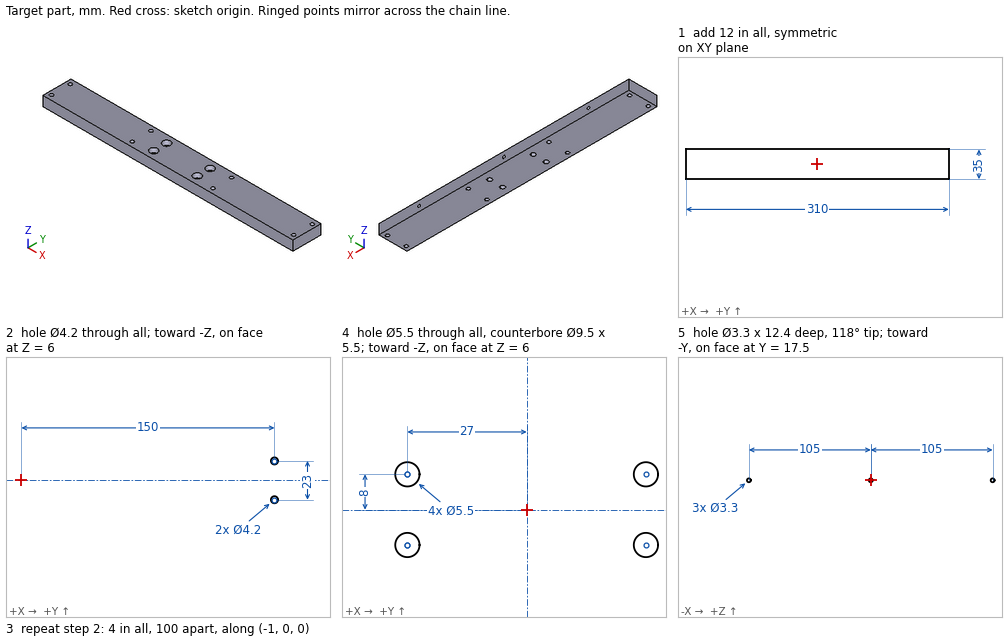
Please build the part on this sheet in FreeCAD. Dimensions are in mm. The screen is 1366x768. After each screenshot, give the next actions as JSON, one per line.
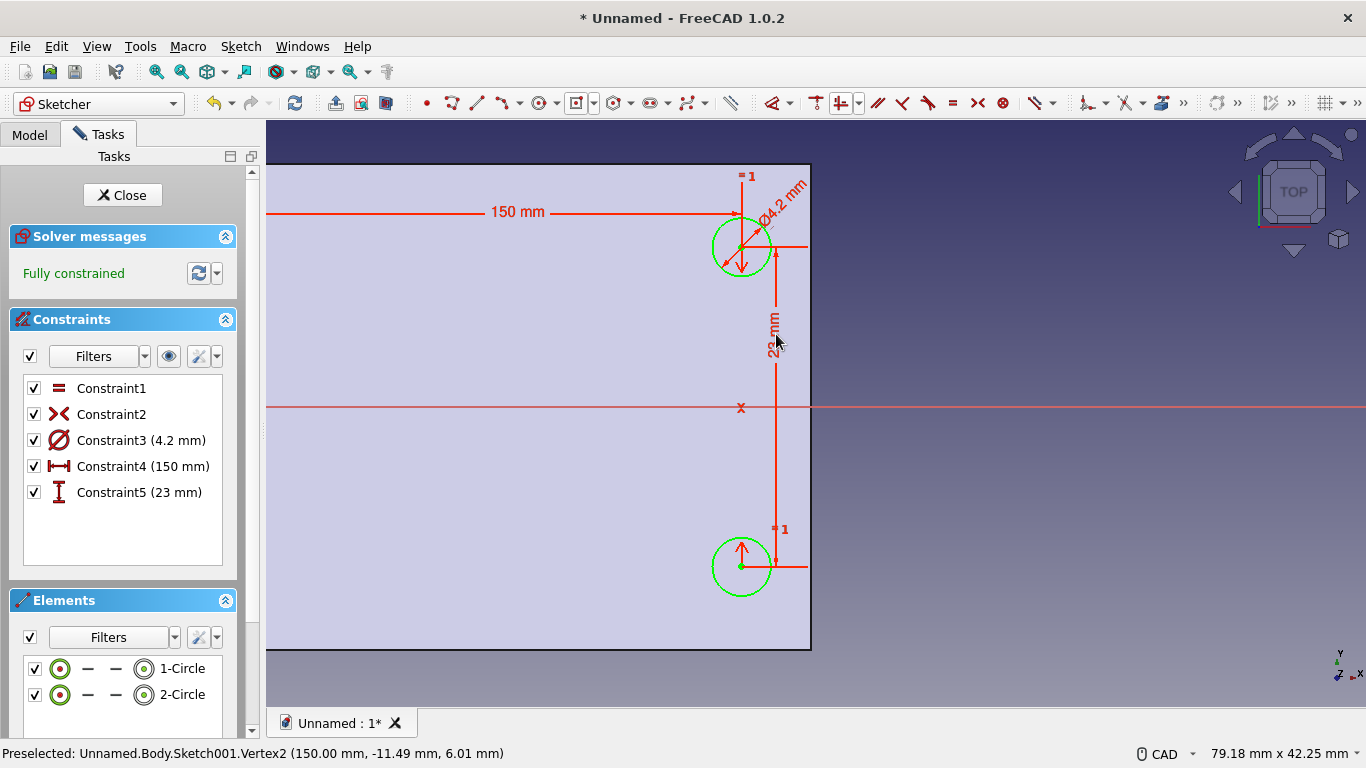
{"action": "left_click", "coordinate": [123, 195]}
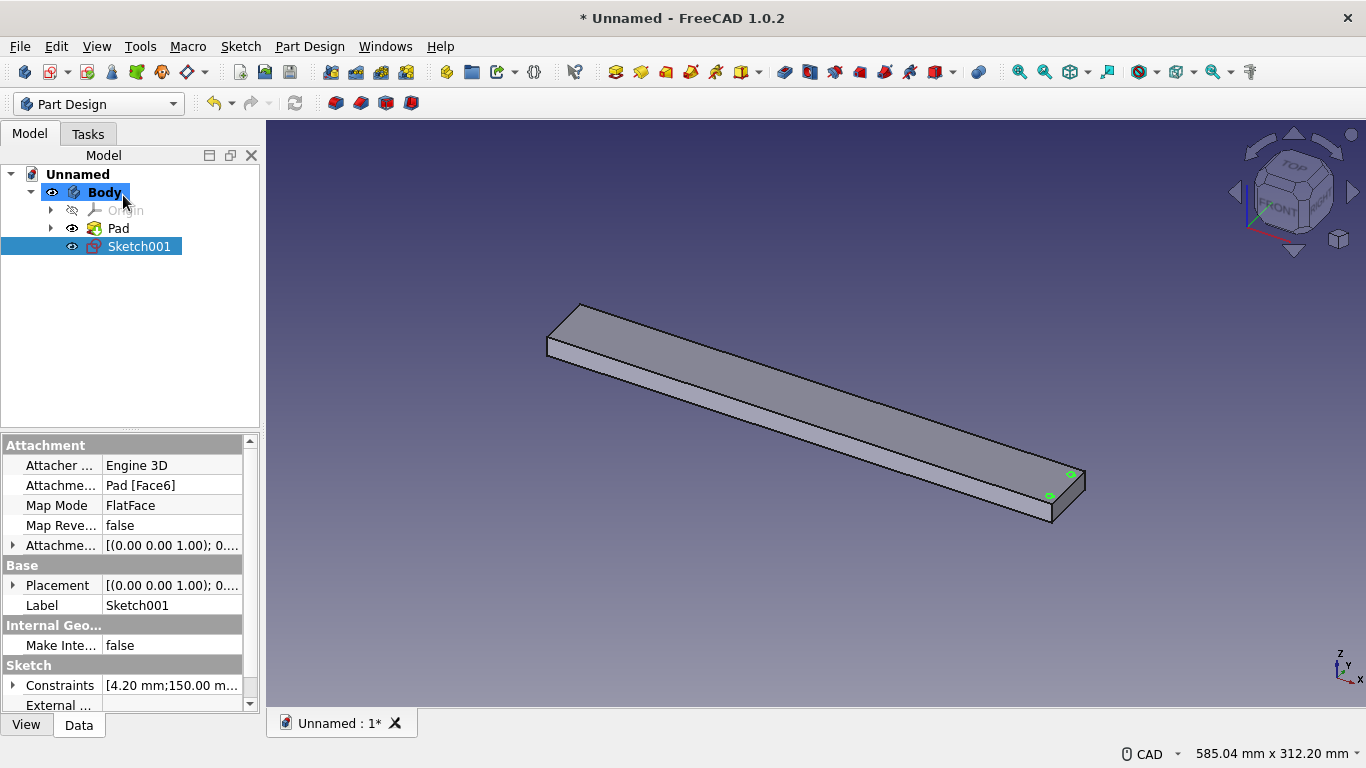
{"action": "left_click", "coordinate": [810, 72]}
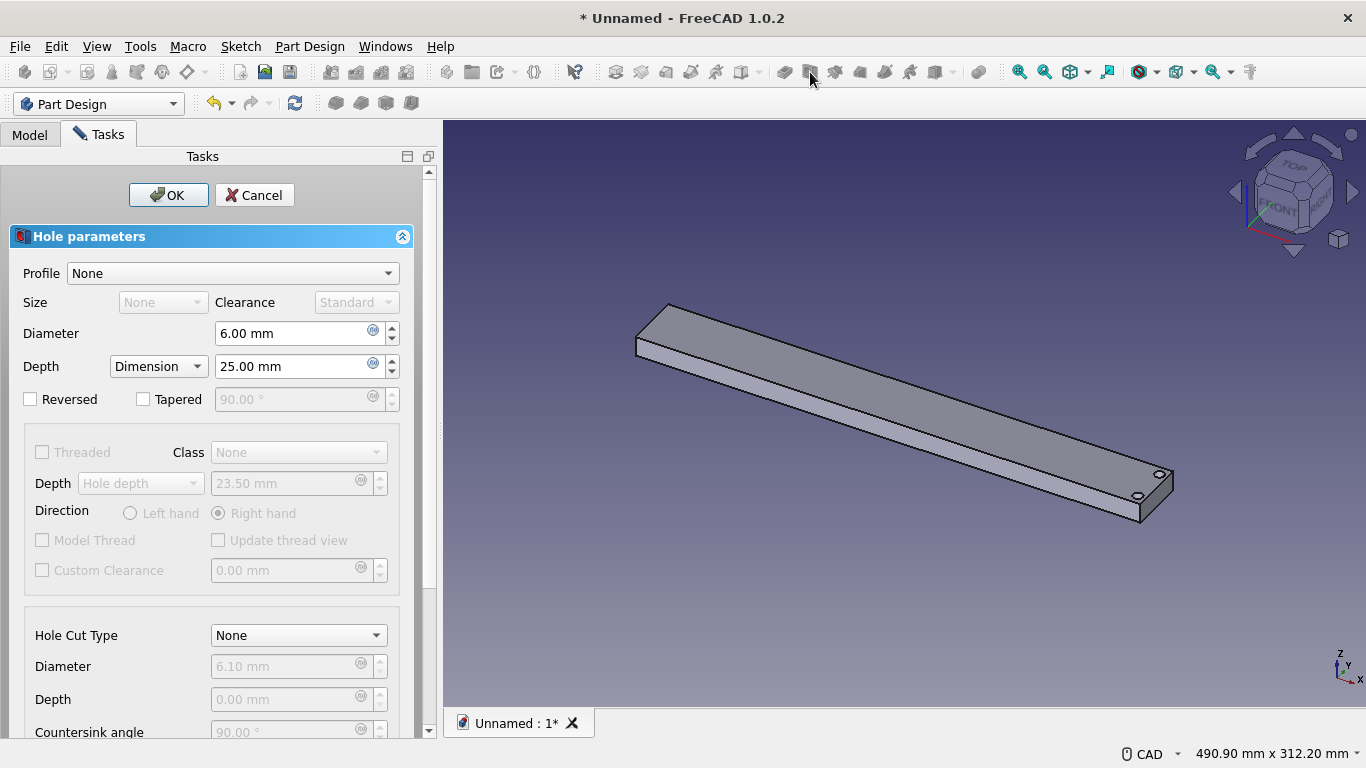
{"action": "triple_click", "coordinate": [300, 334]}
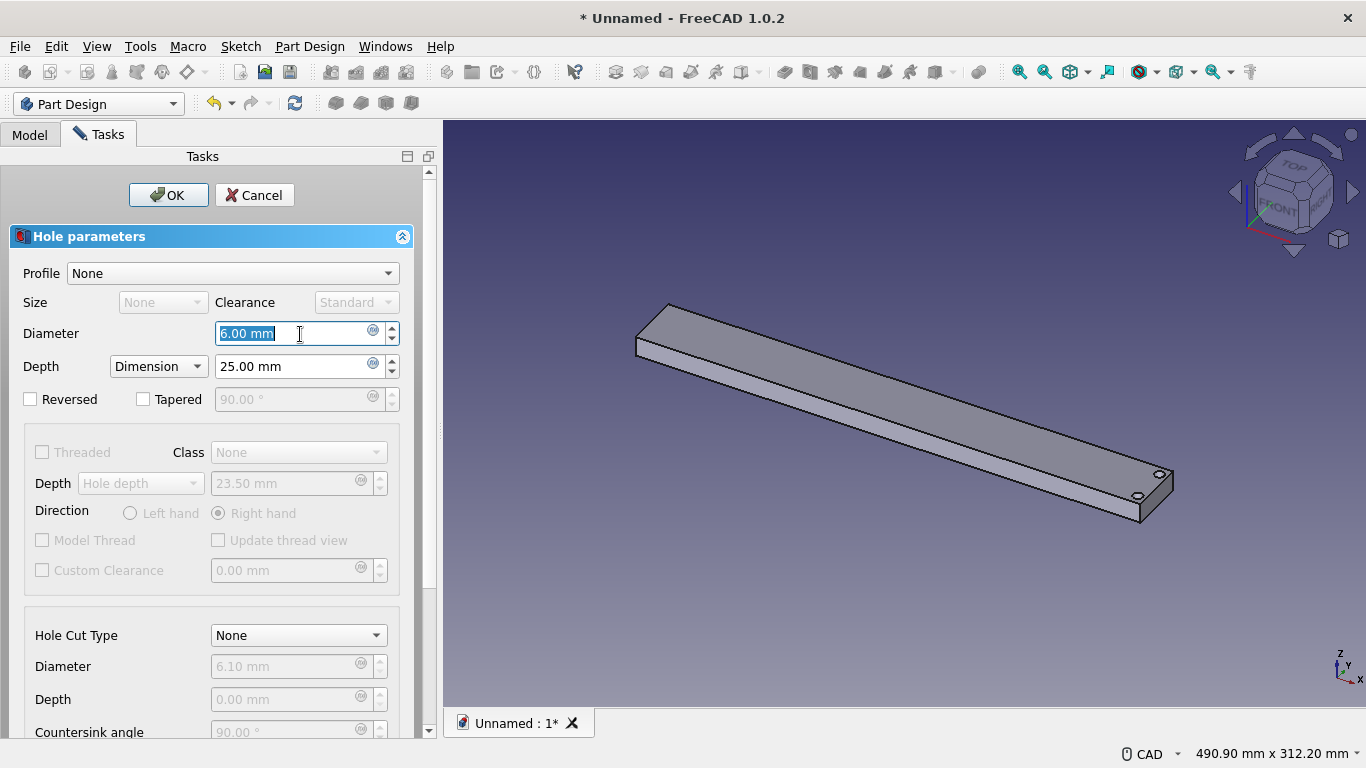
{"action": "type", "text": "4.2"}
{"action": "key", "text": "Tab"}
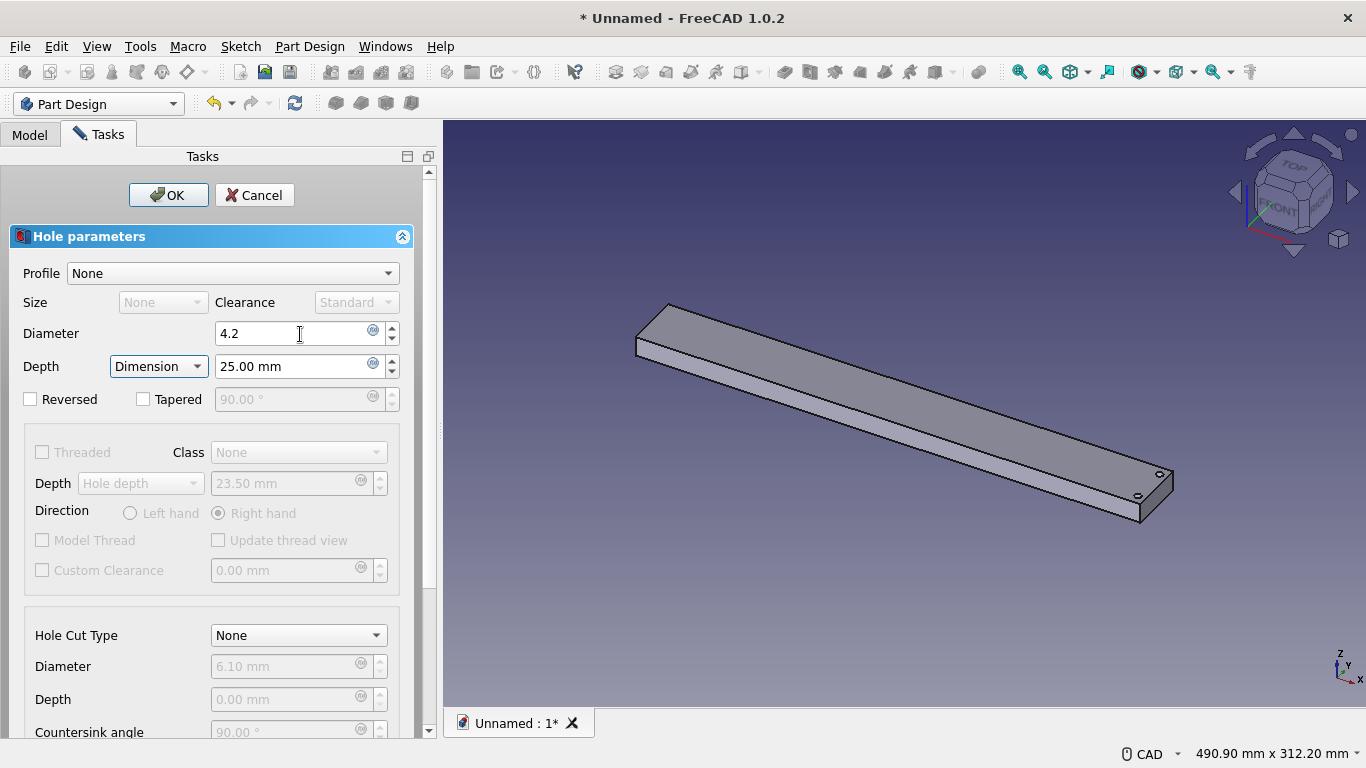
{"action": "left_click", "coordinate": [160, 366]}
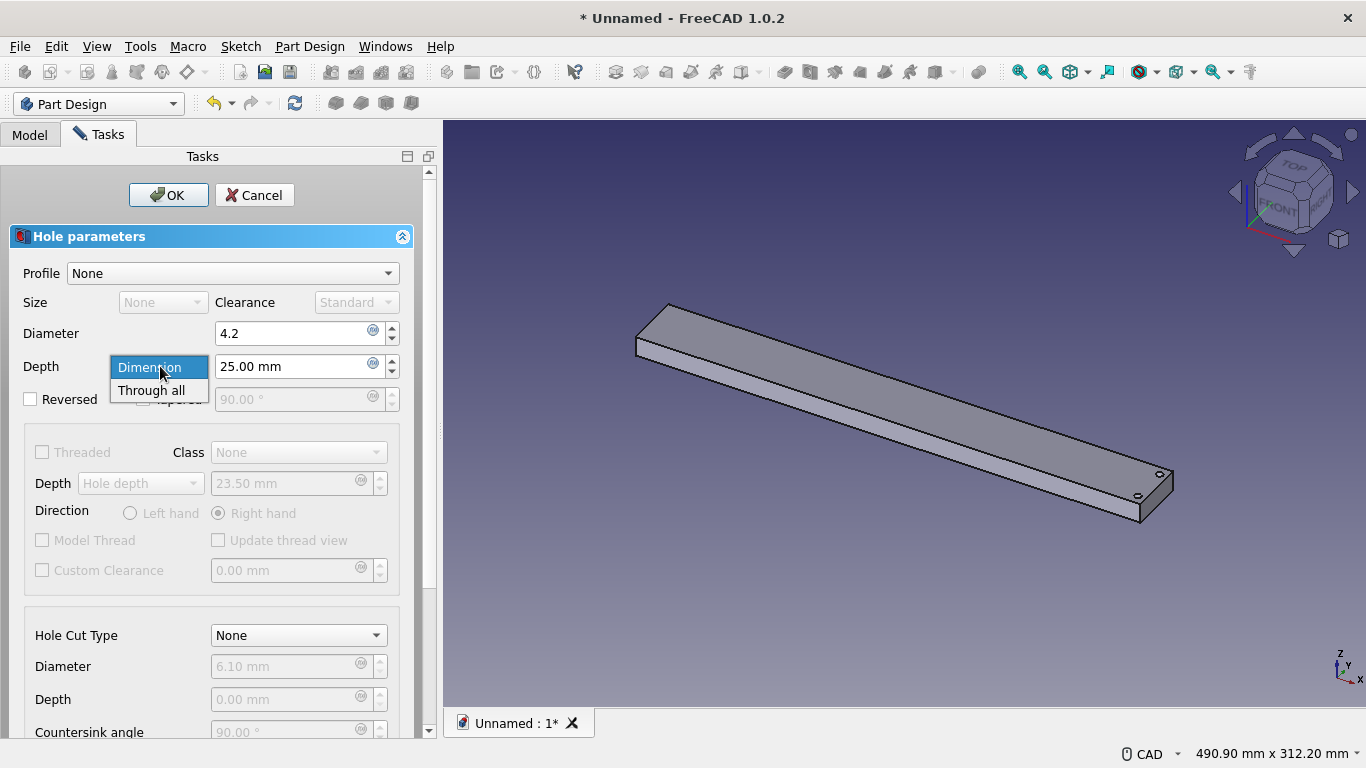
{"action": "left_click", "coordinate": [158, 390]}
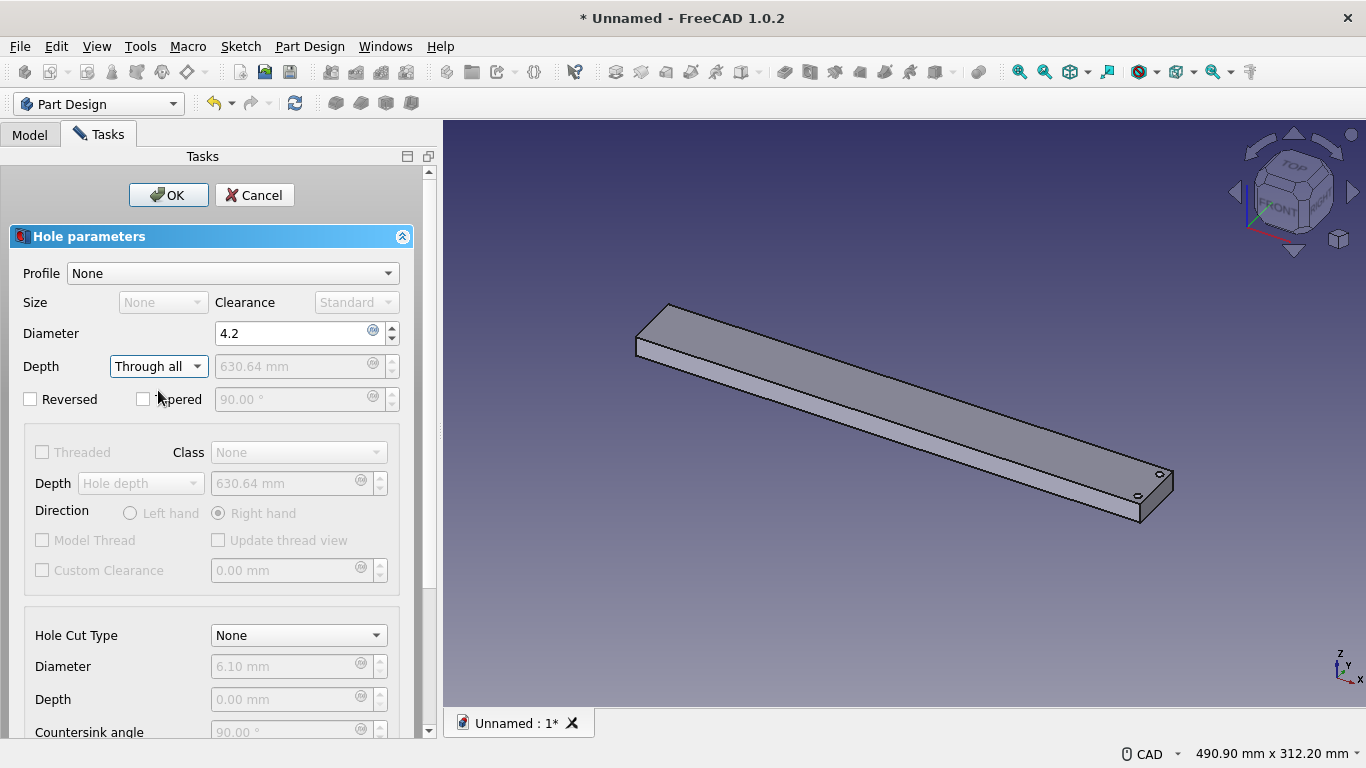
{"action": "left_click", "coordinate": [169, 195]}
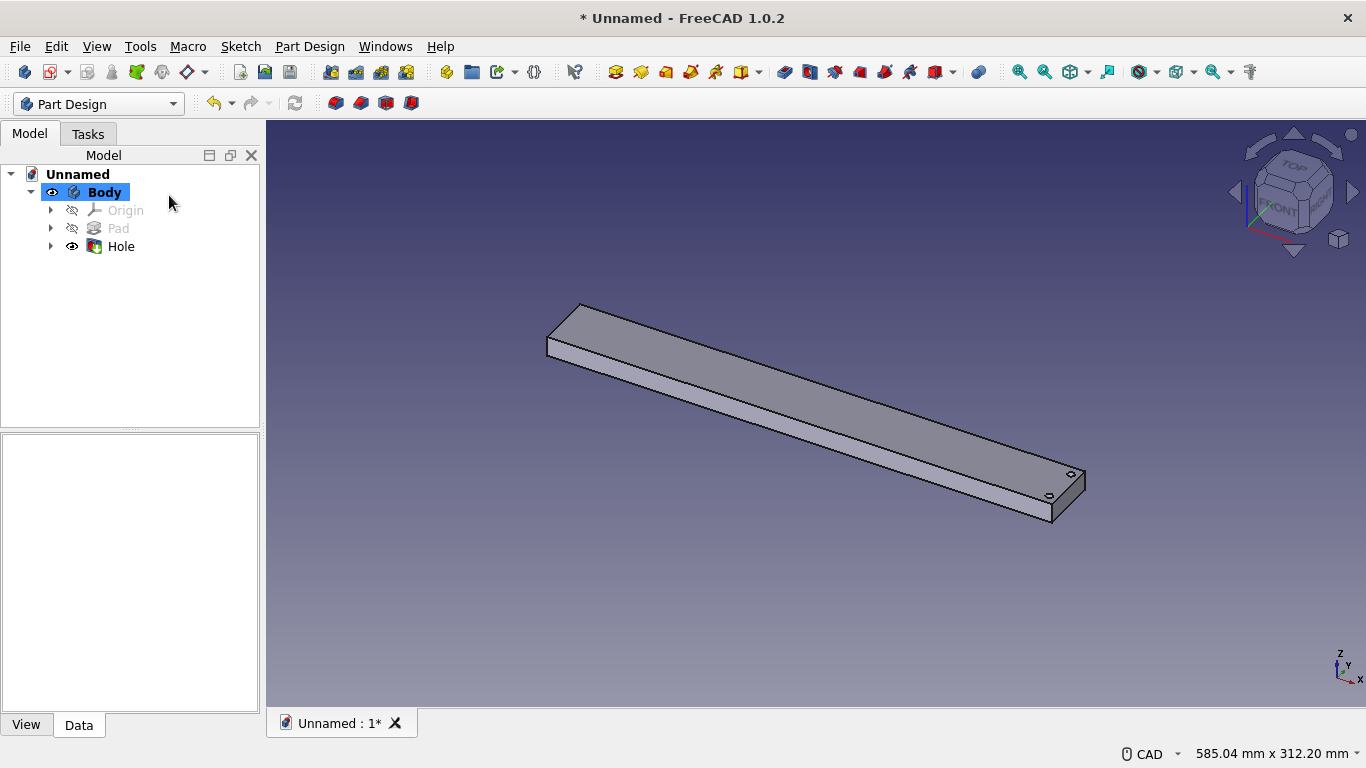
{"action": "left_click", "coordinate": [117, 246]}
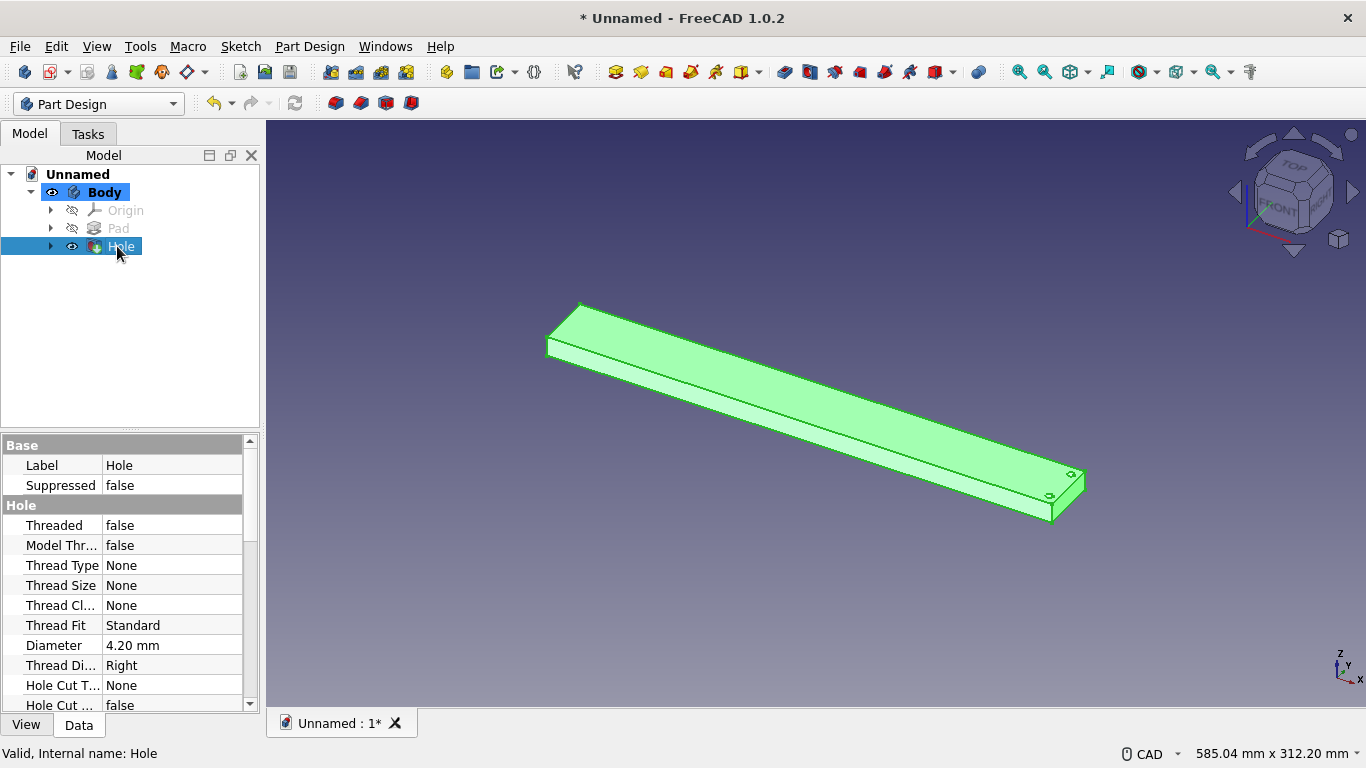
{"action": "left_click", "coordinate": [356, 72]}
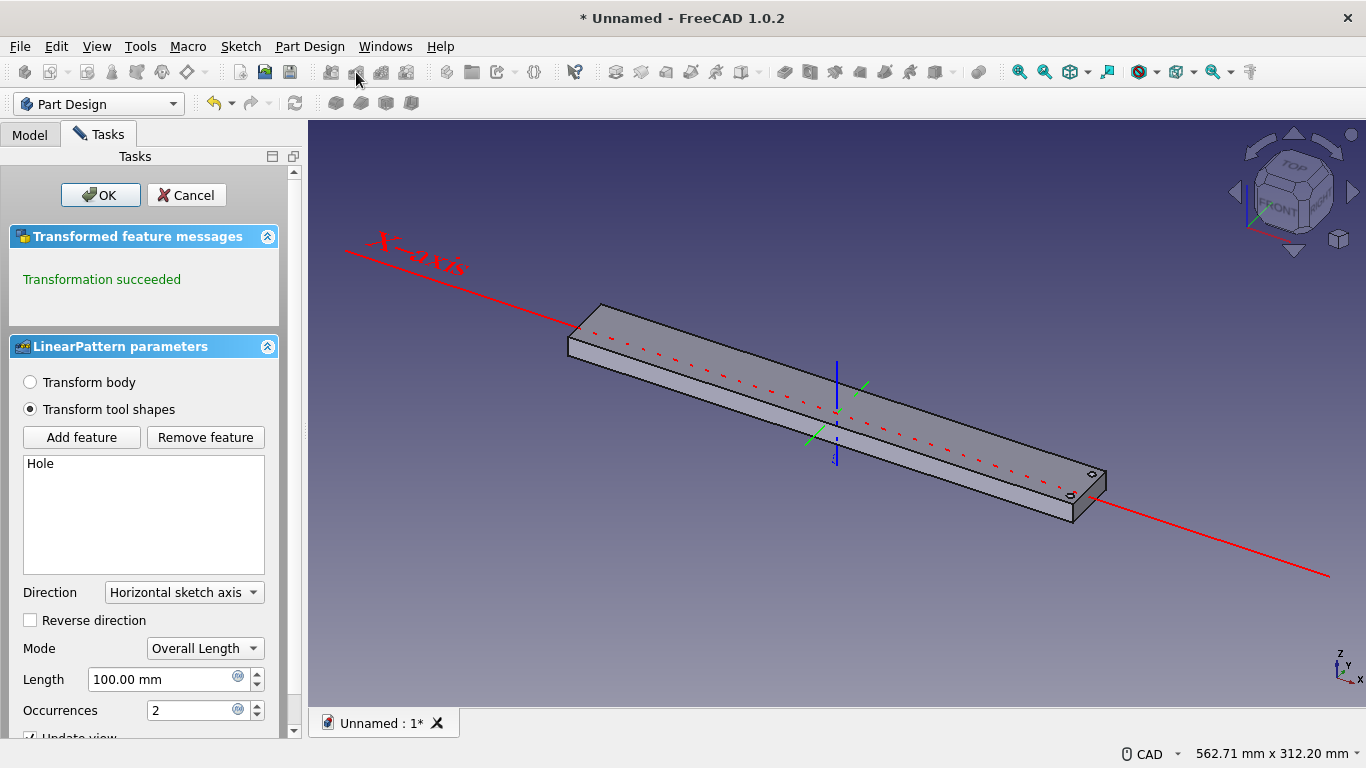
{"action": "left_click", "coordinate": [185, 592]}